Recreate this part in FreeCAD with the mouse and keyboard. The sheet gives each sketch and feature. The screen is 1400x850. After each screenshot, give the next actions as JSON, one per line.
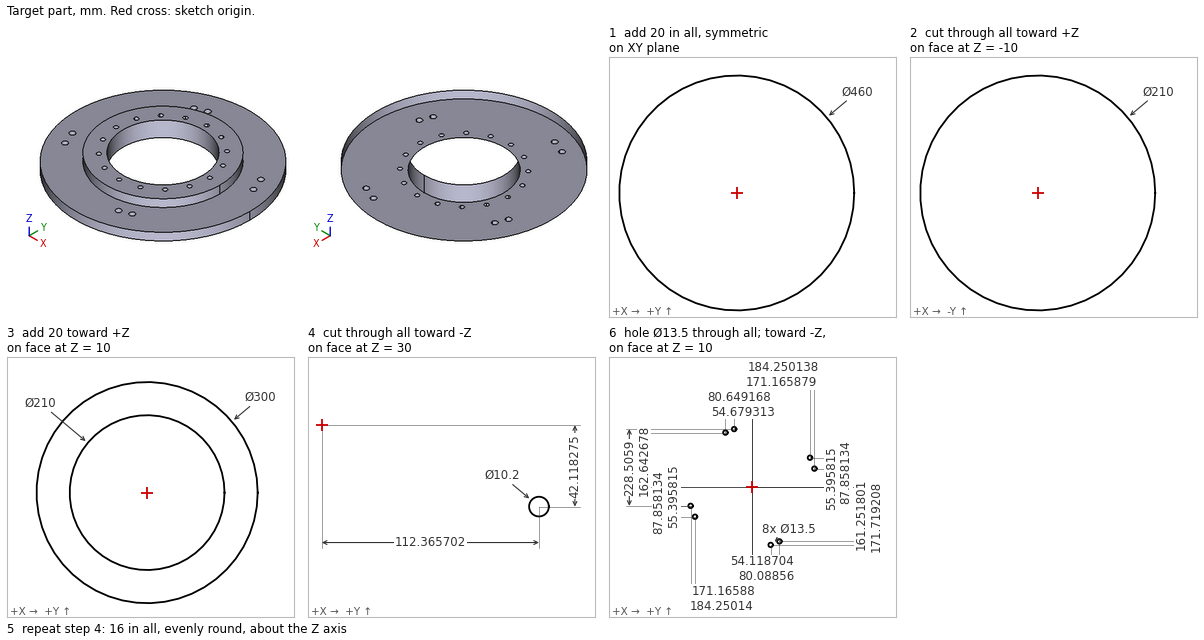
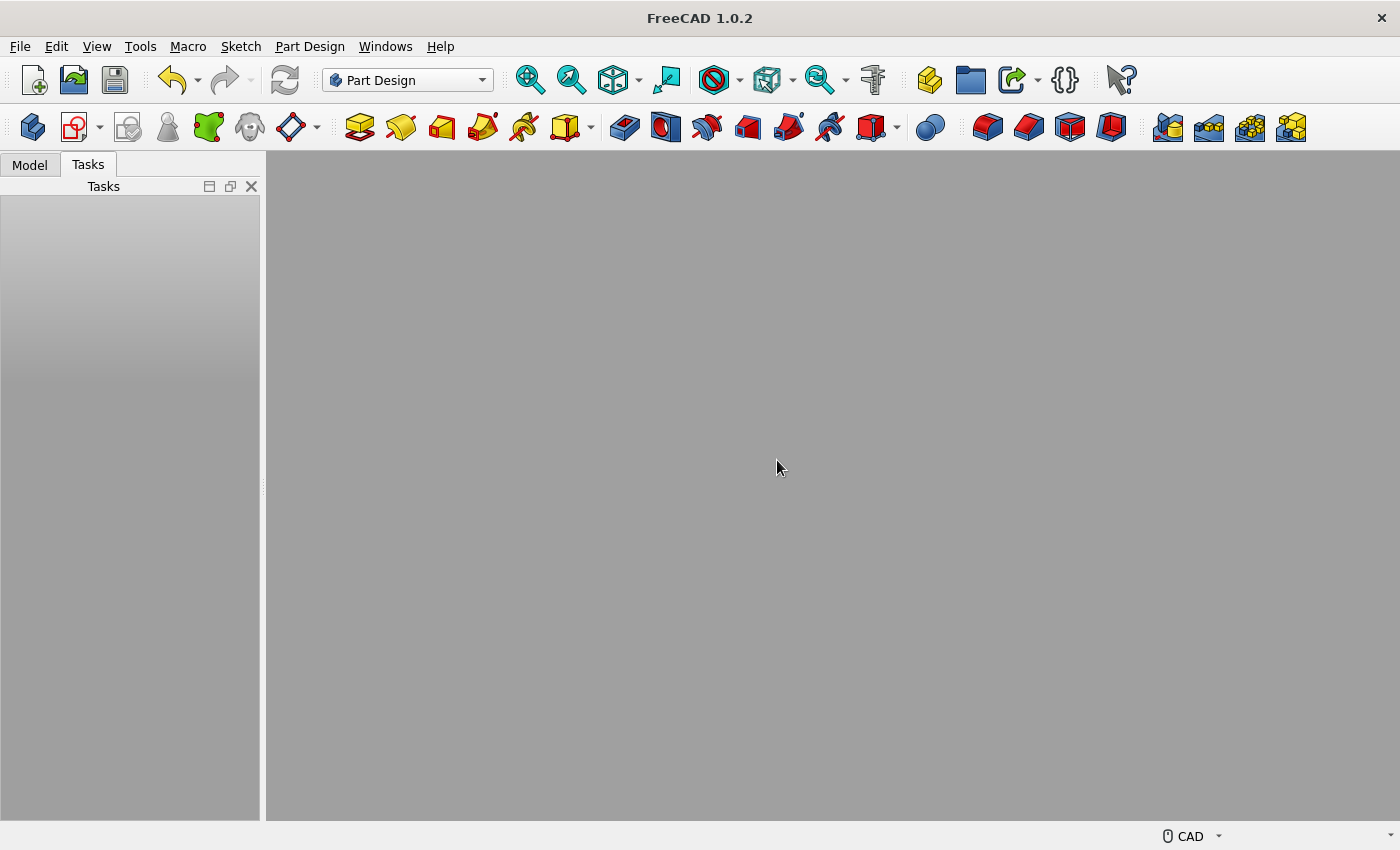
{"action": "left_click", "coordinate": [33, 80]}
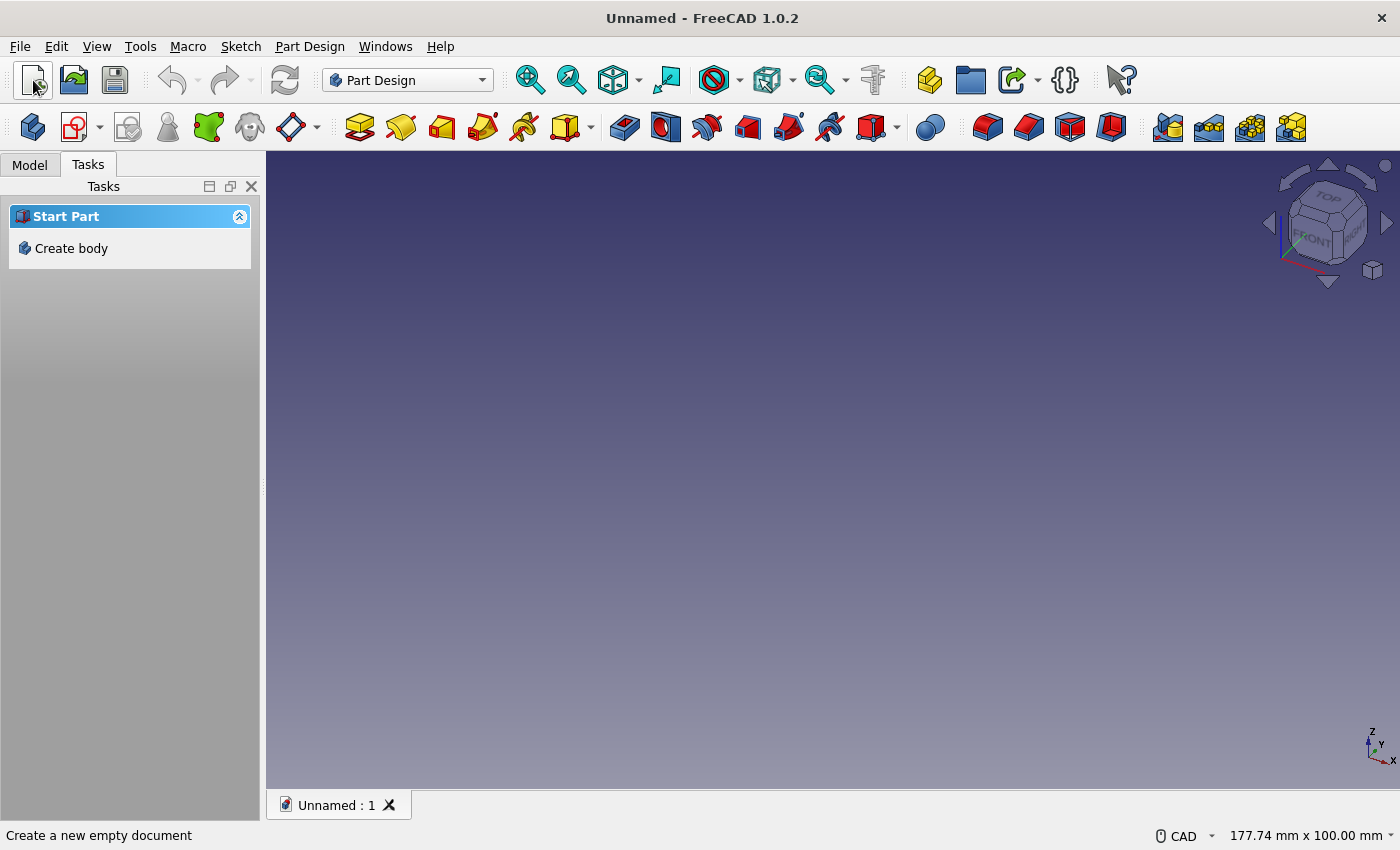
{"action": "left_click", "coordinate": [74, 128]}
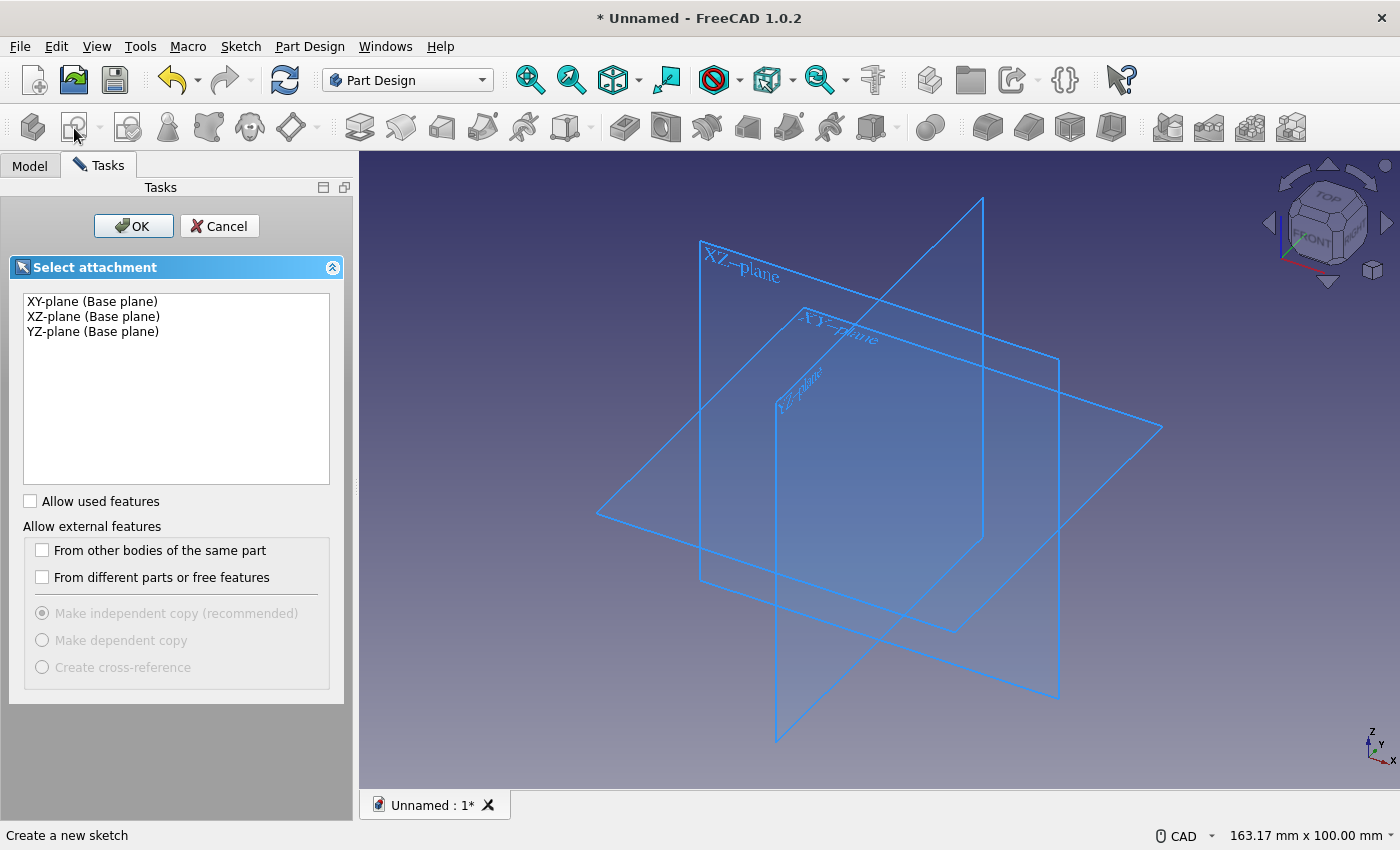
{"action": "left_click", "coordinate": [84, 302]}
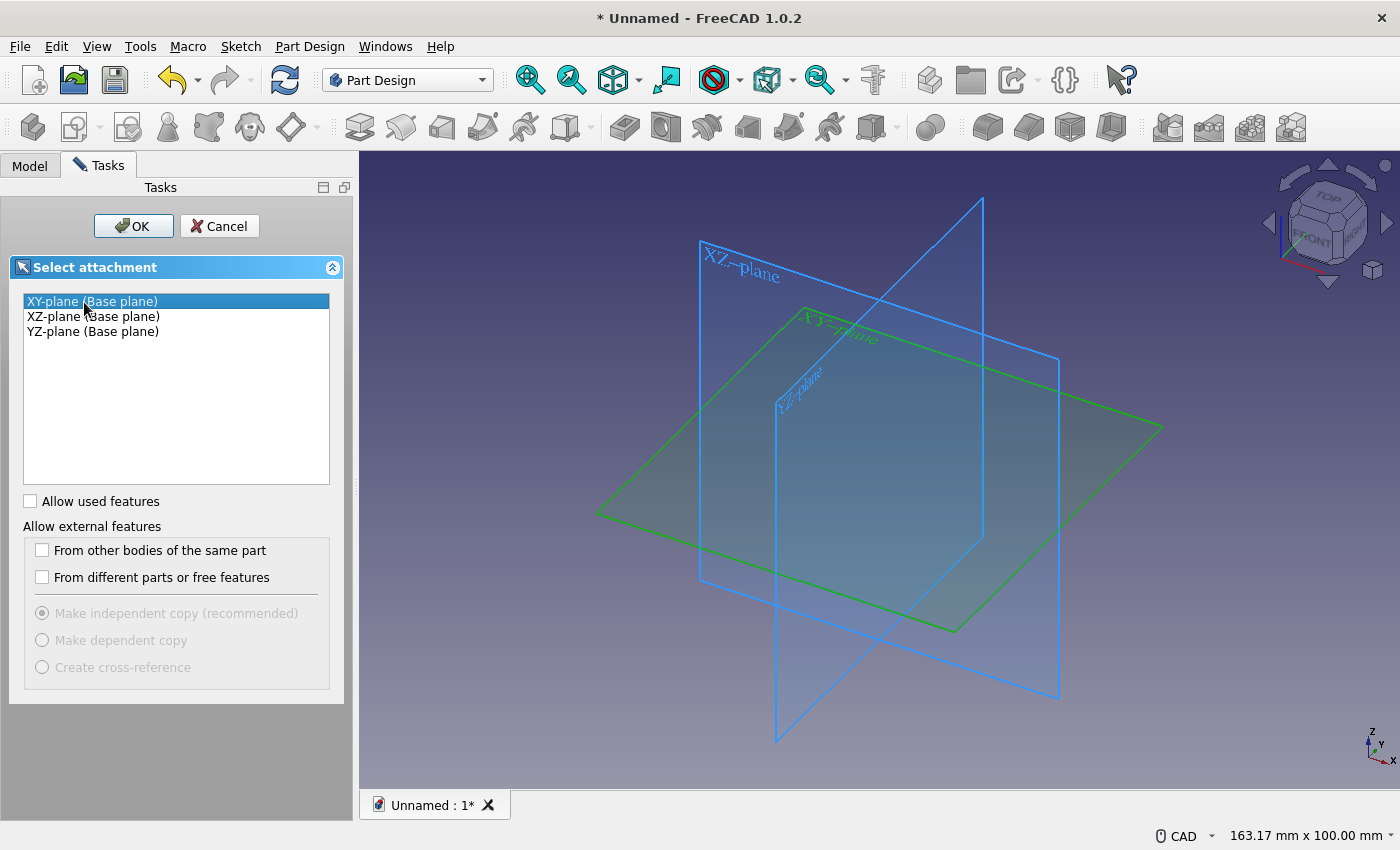
{"action": "left_click", "coordinate": [134, 226]}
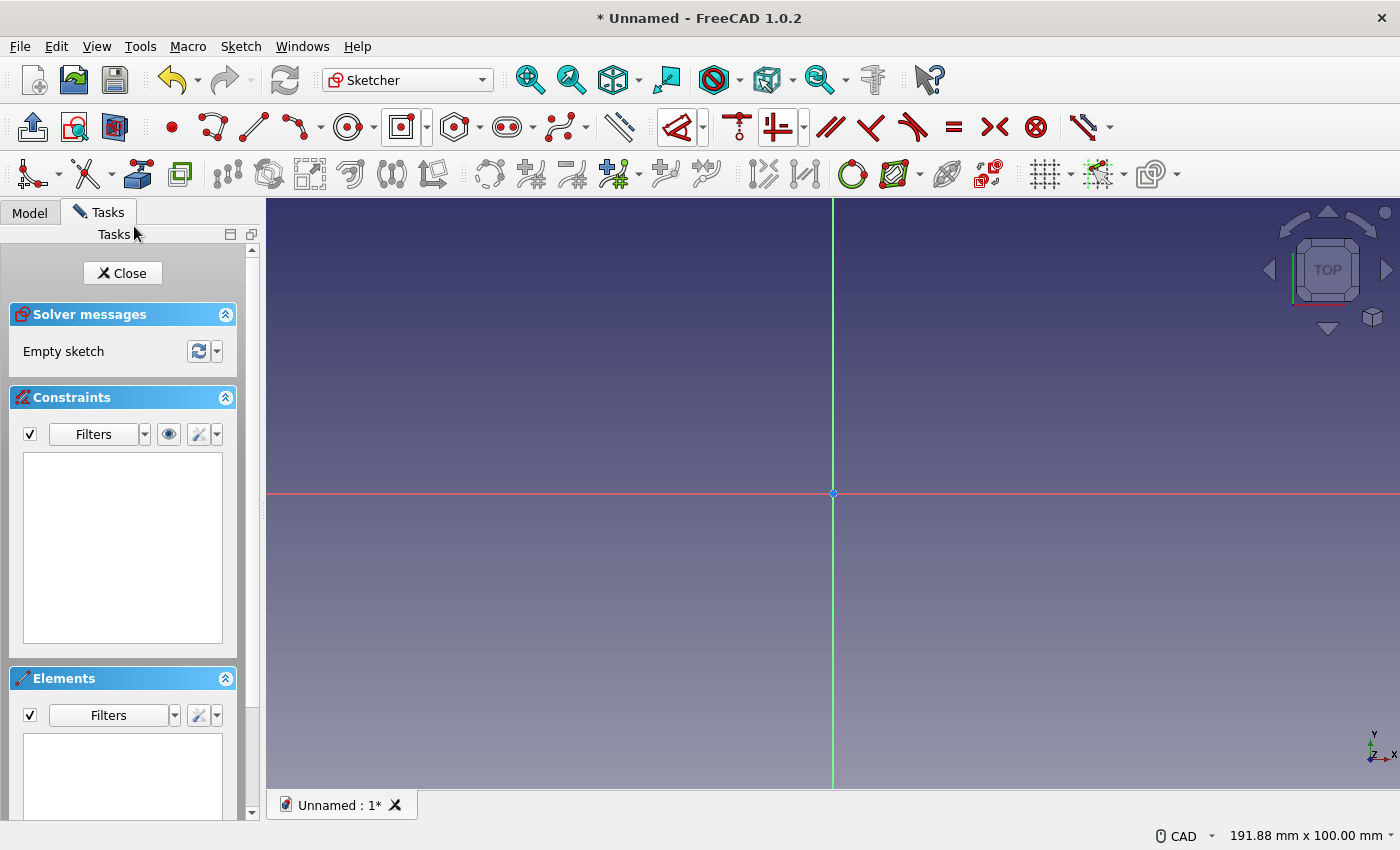
{"action": "scroll", "coordinate": [754, 494], "scroll_direction": "down", "scroll_amount": 10}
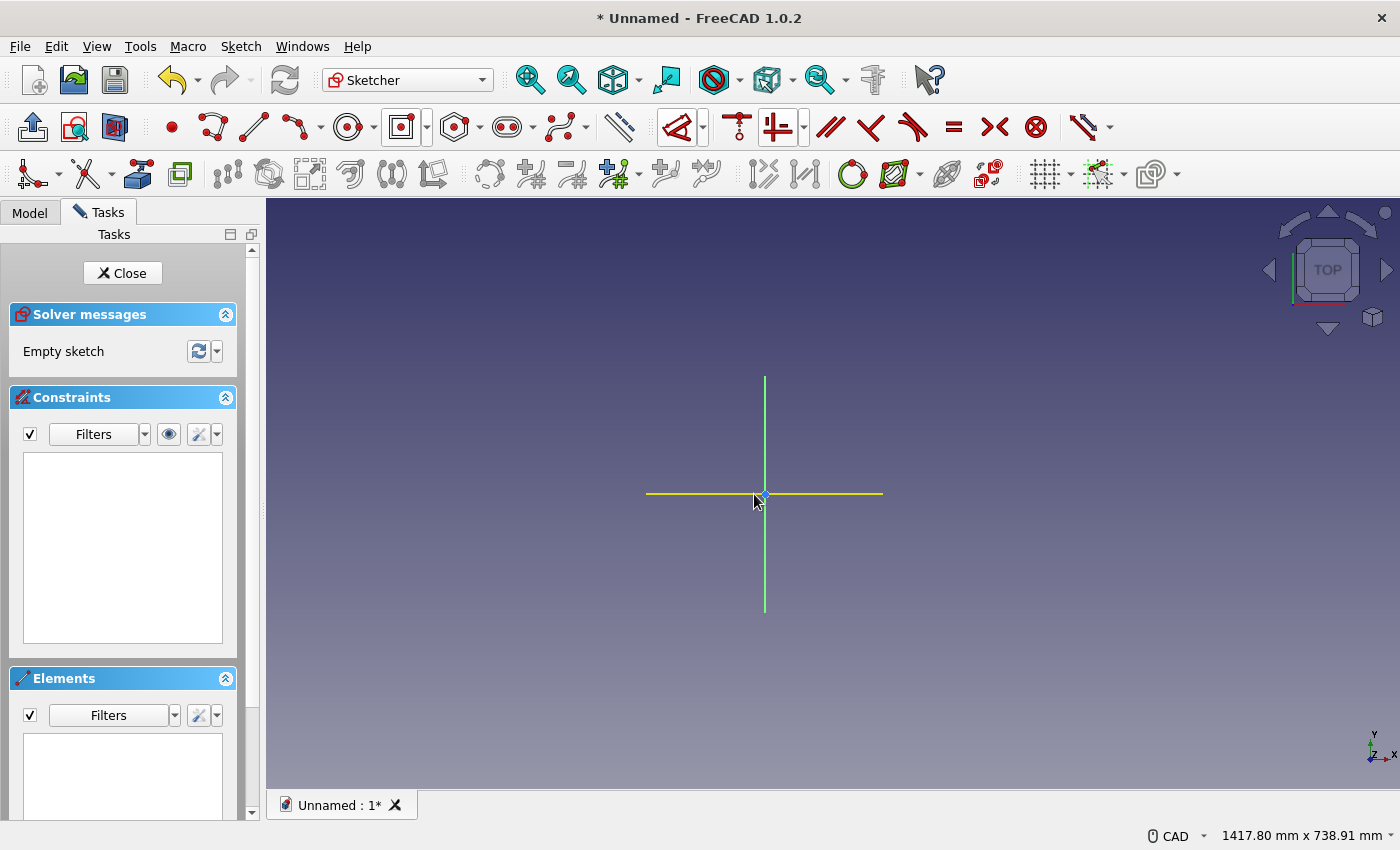
{"action": "key", "text": "g c"}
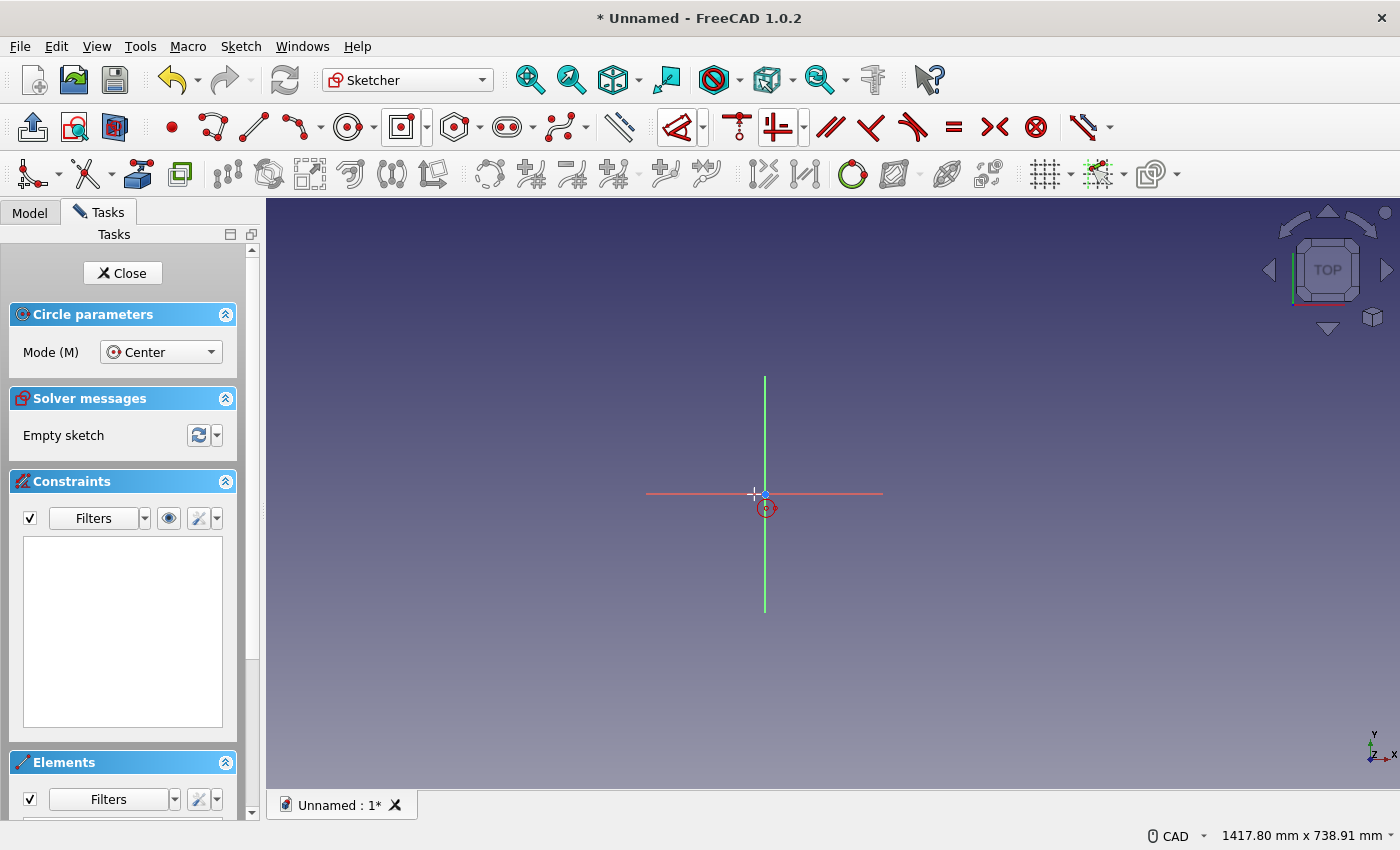
{"action": "left_click", "coordinate": [765, 494]}
{"action": "mouse_move", "coordinate": [895, 364]}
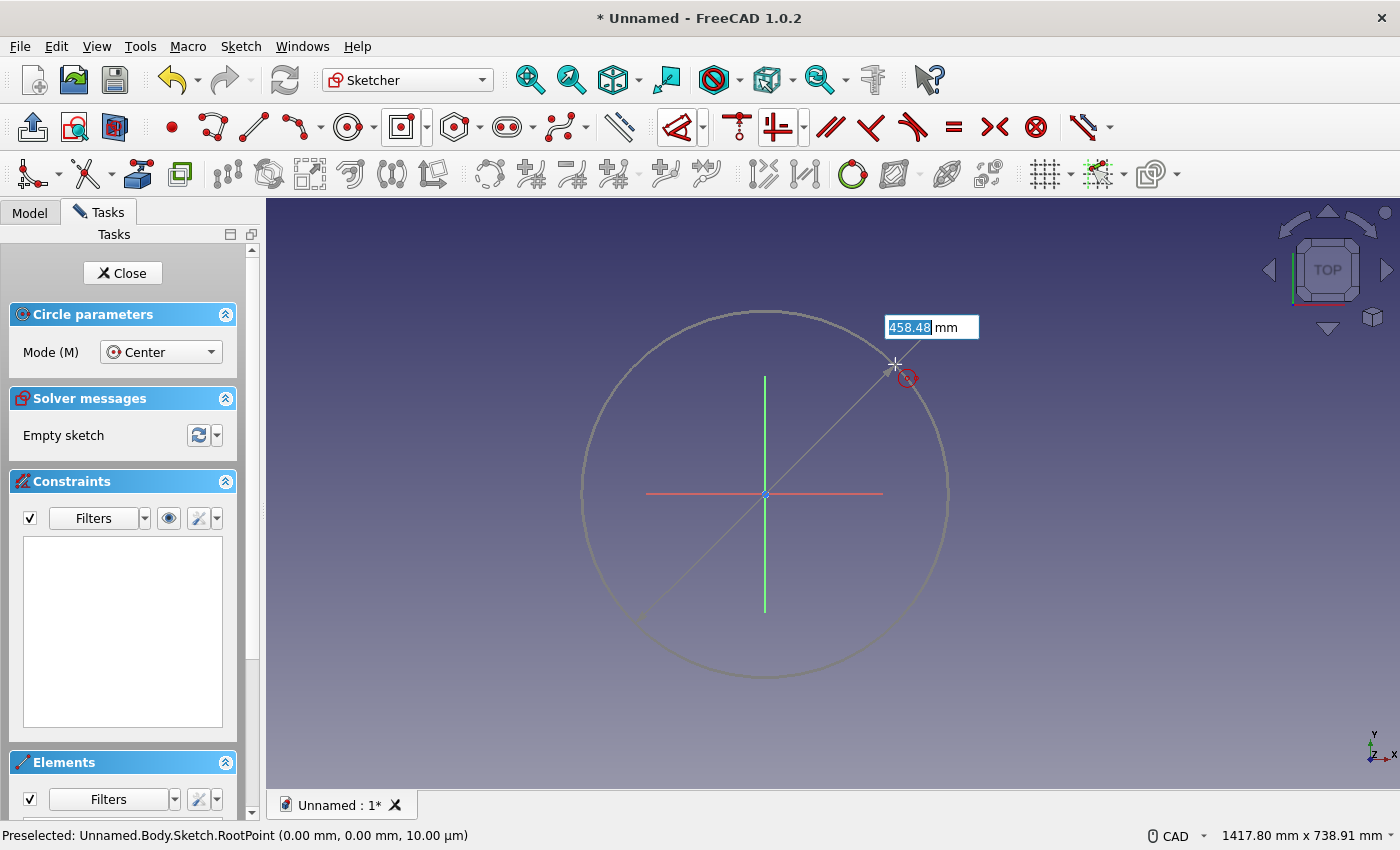
{"action": "type", "text": "460"}
{"action": "key", "text": "Return"}
{"action": "key", "text": "Escape"}